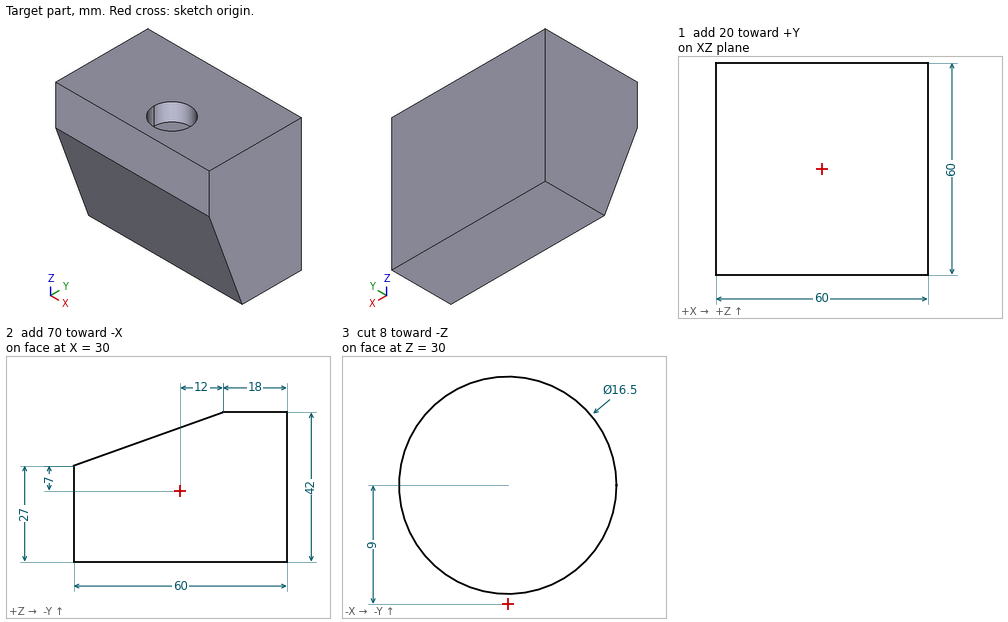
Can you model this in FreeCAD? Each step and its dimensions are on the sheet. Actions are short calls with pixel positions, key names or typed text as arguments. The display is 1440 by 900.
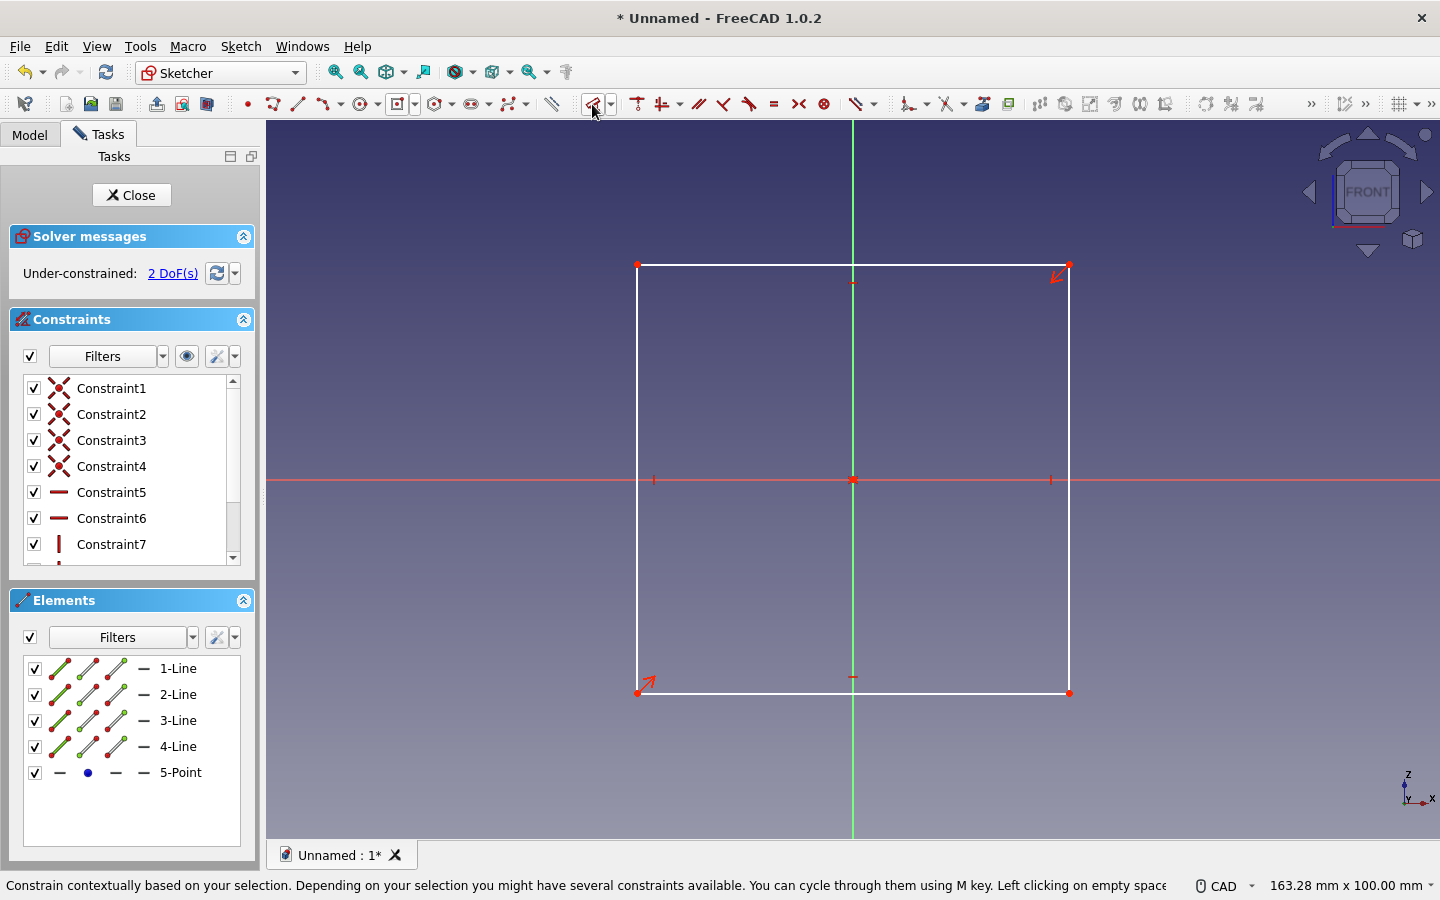
click(767, 694)
click(754, 728)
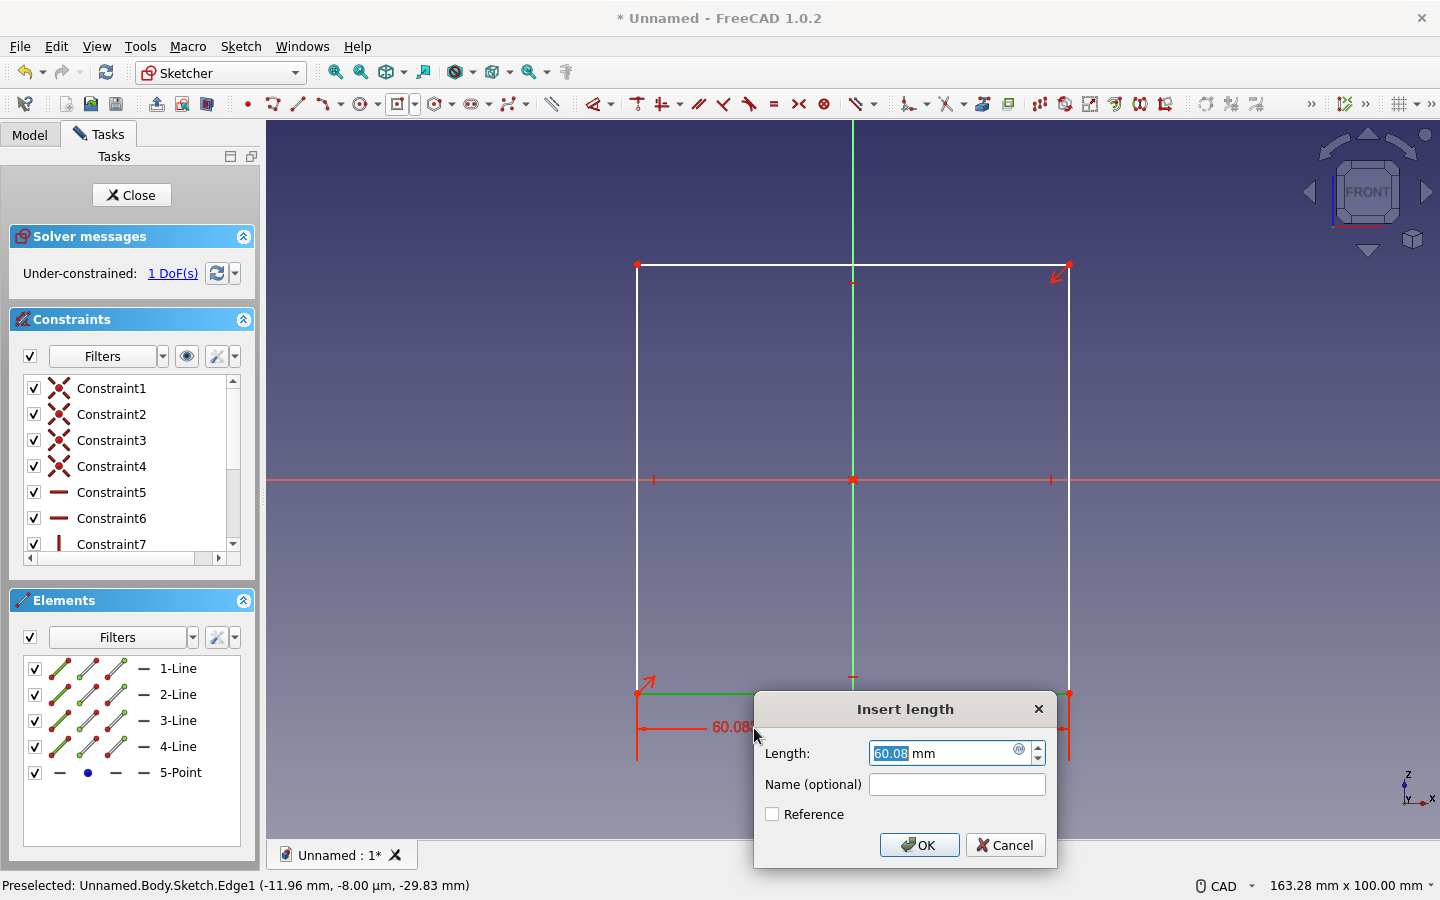
text(60)
key(Return)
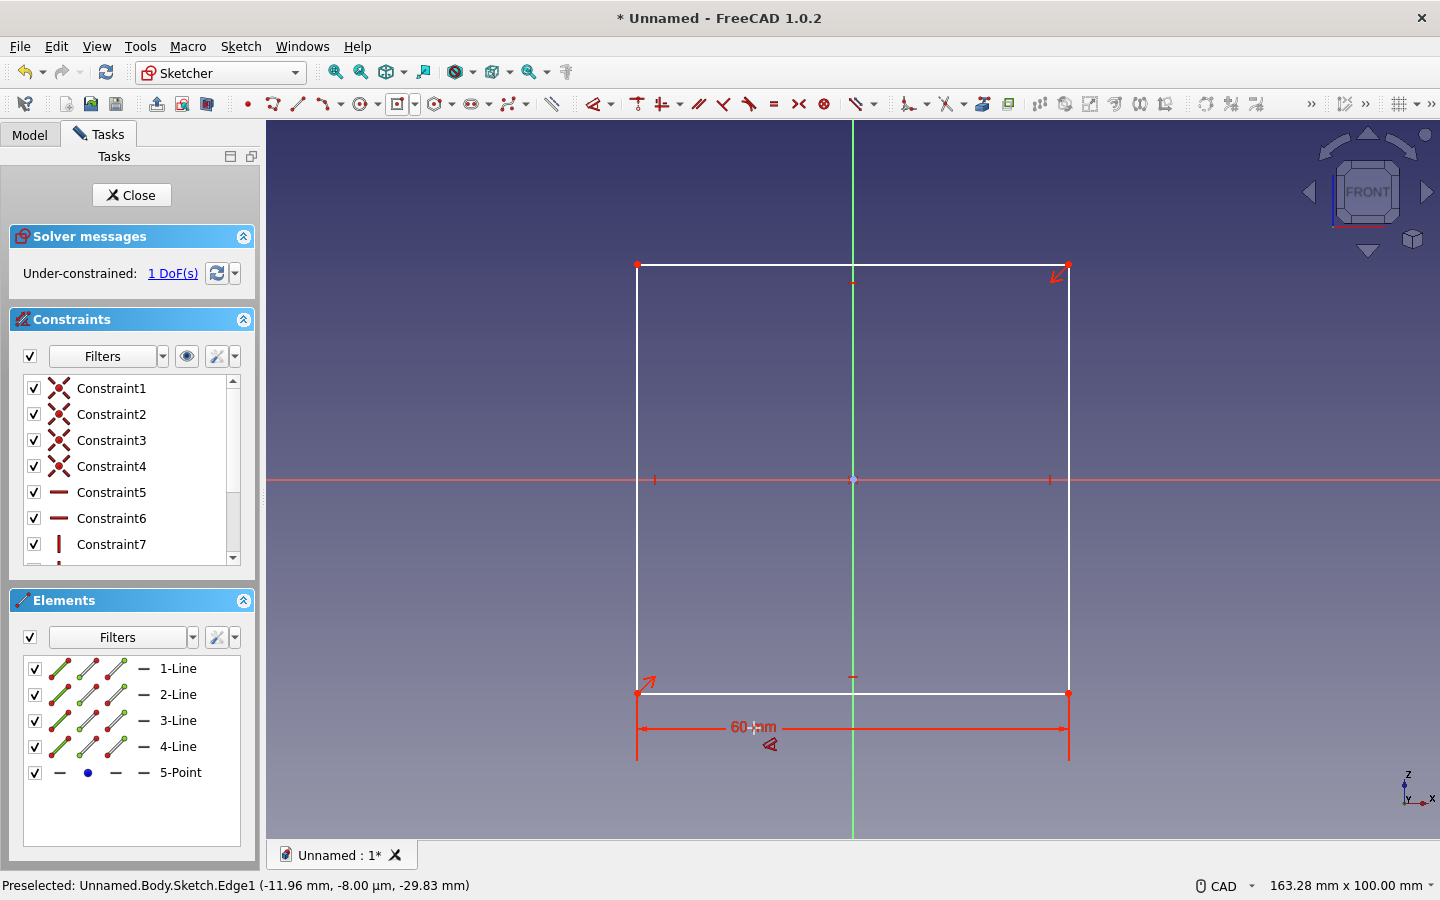
click(1069, 565)
click(1103, 381)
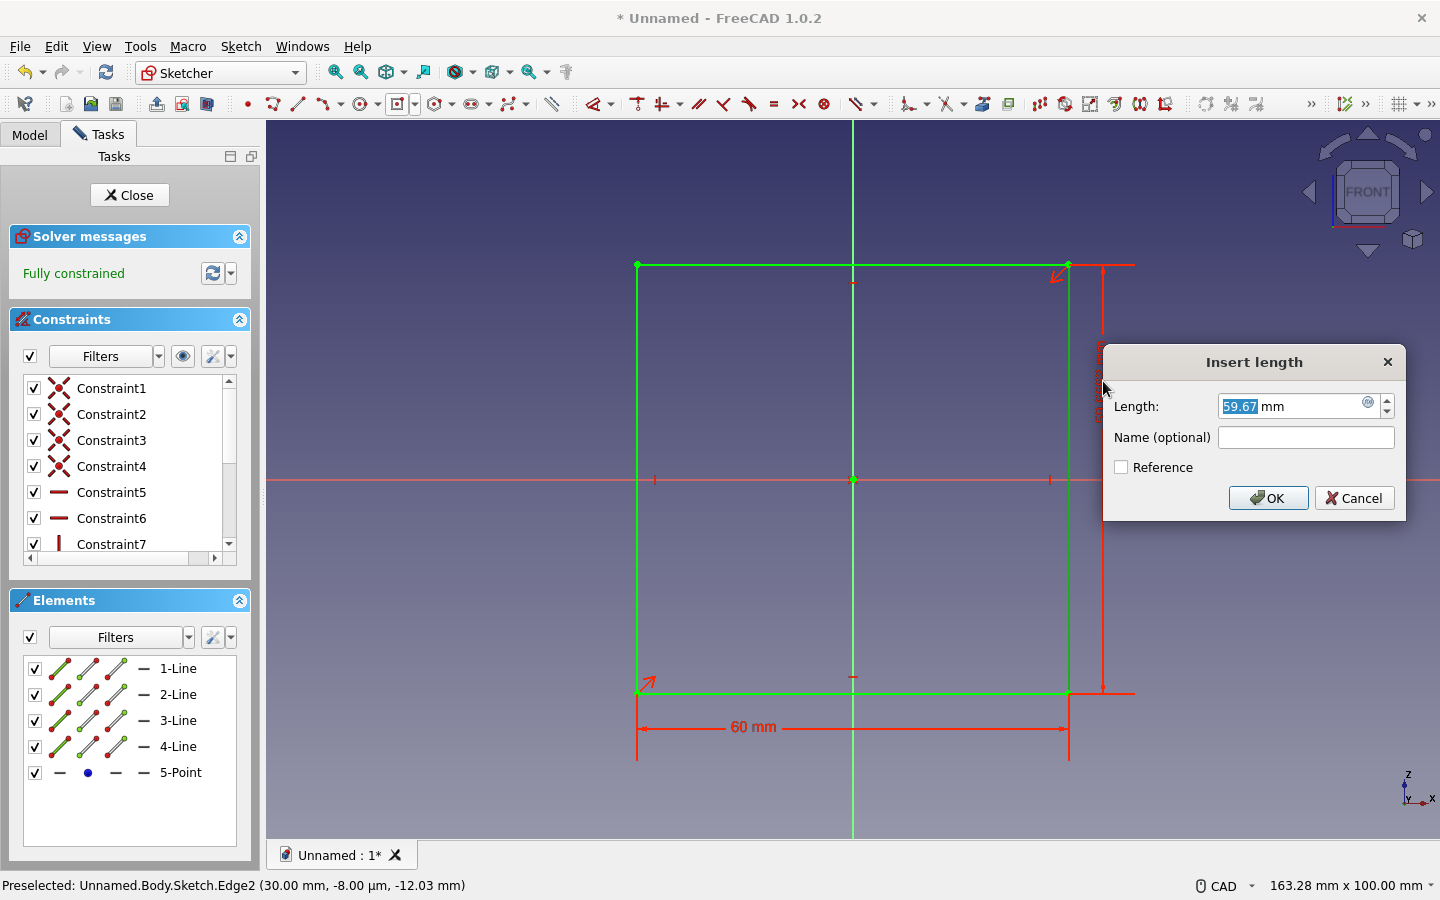
text(60)
key(Return)
key(Escape)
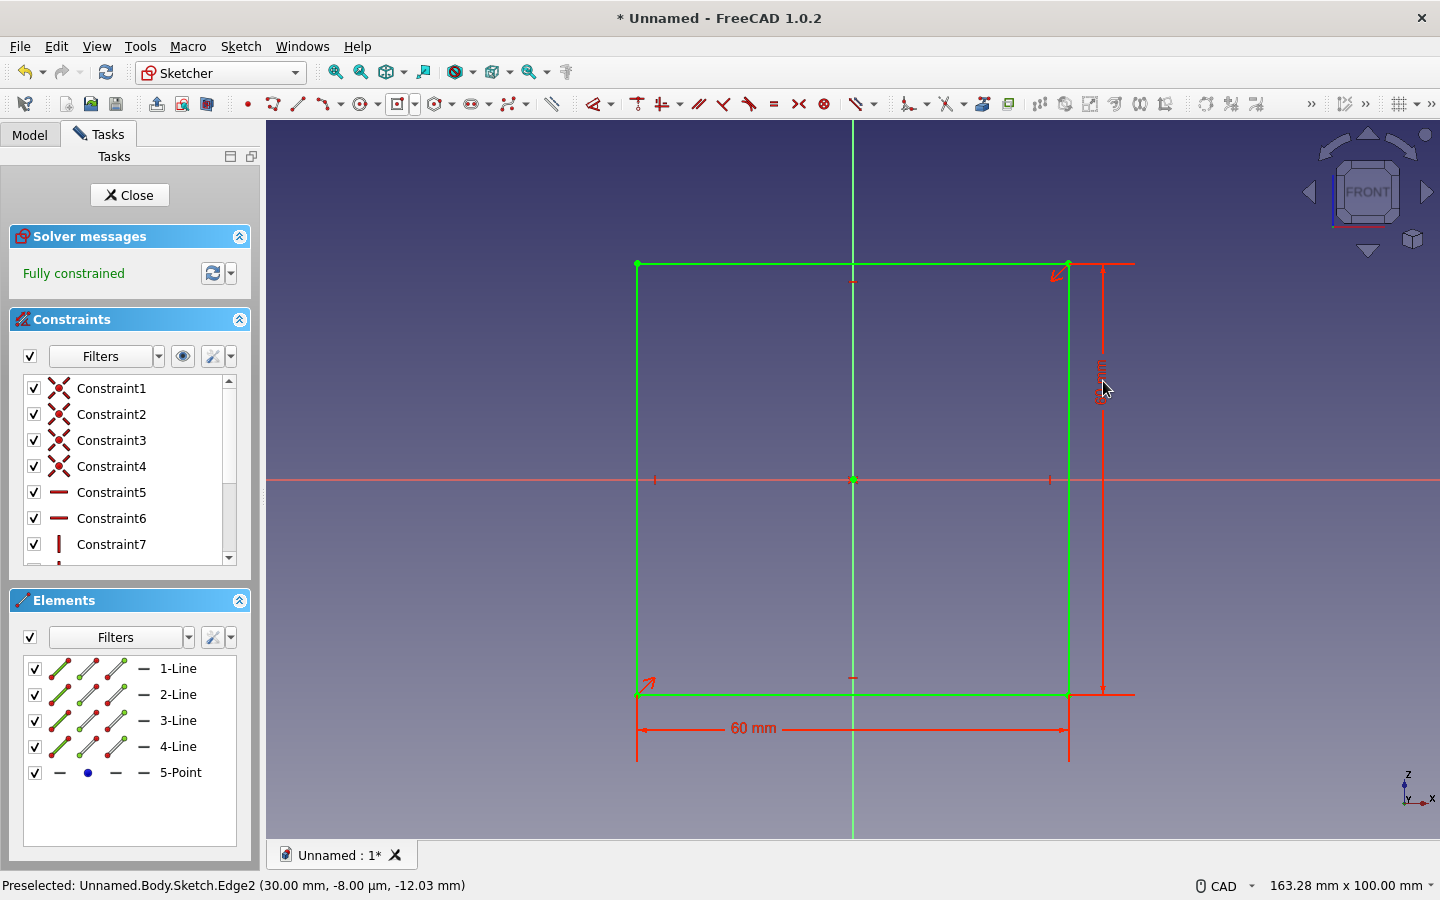
click(130, 195)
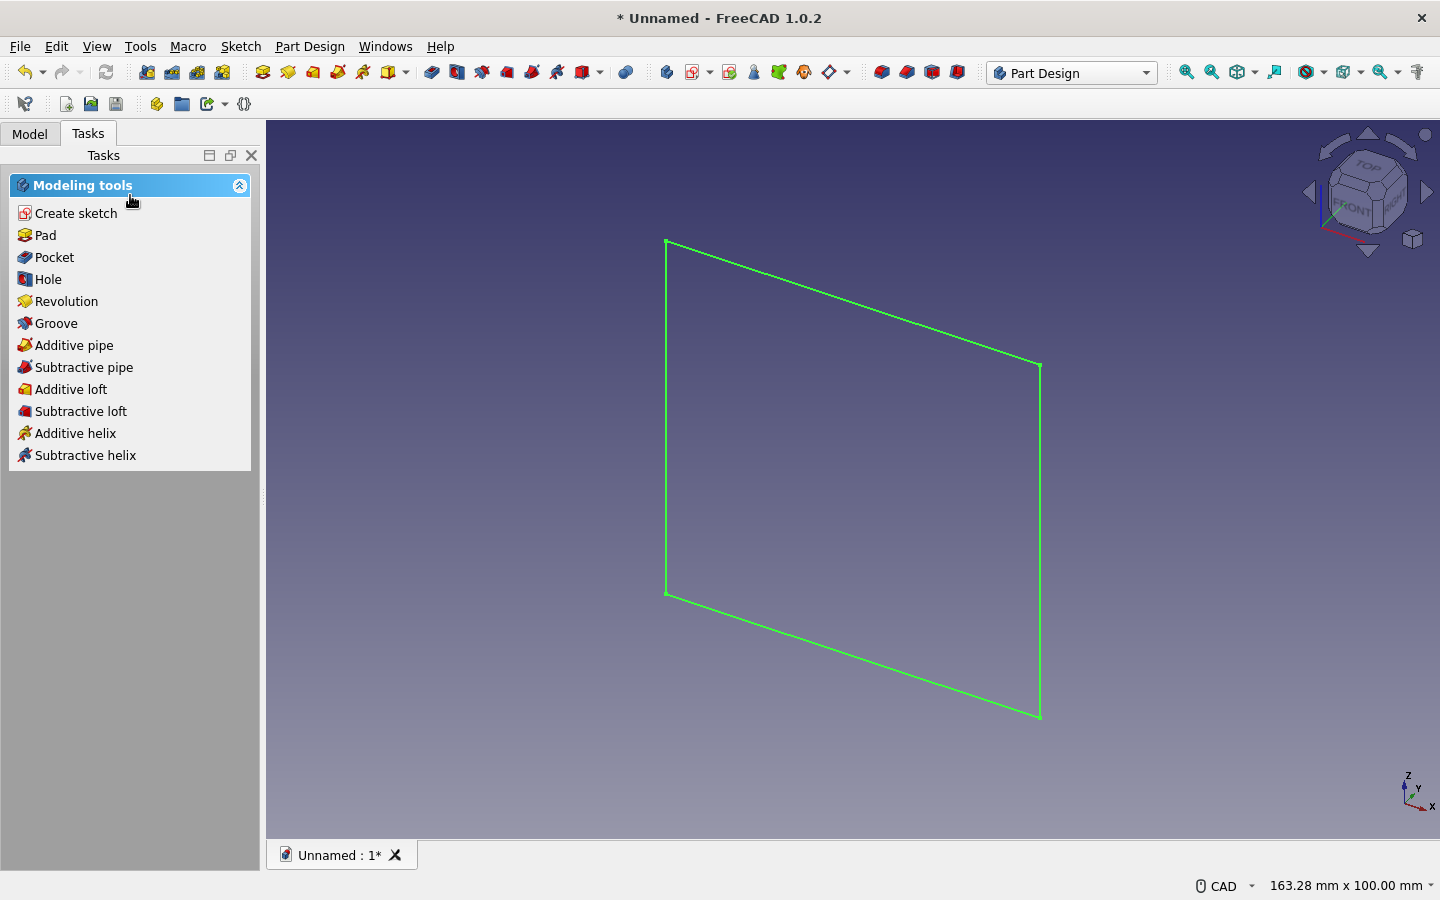
click(263, 72)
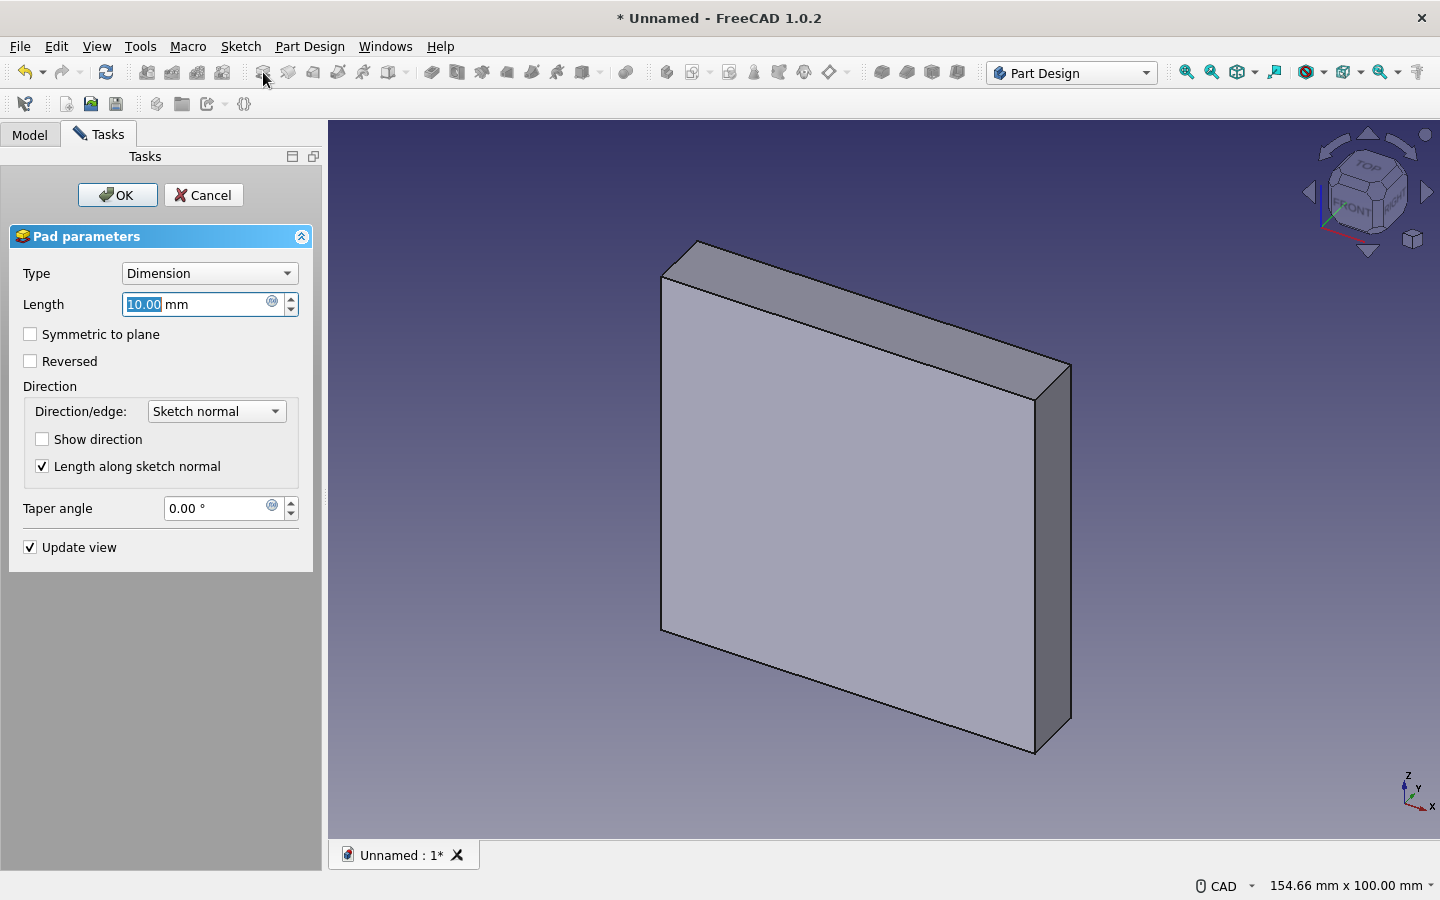
text(20)
key(Tab)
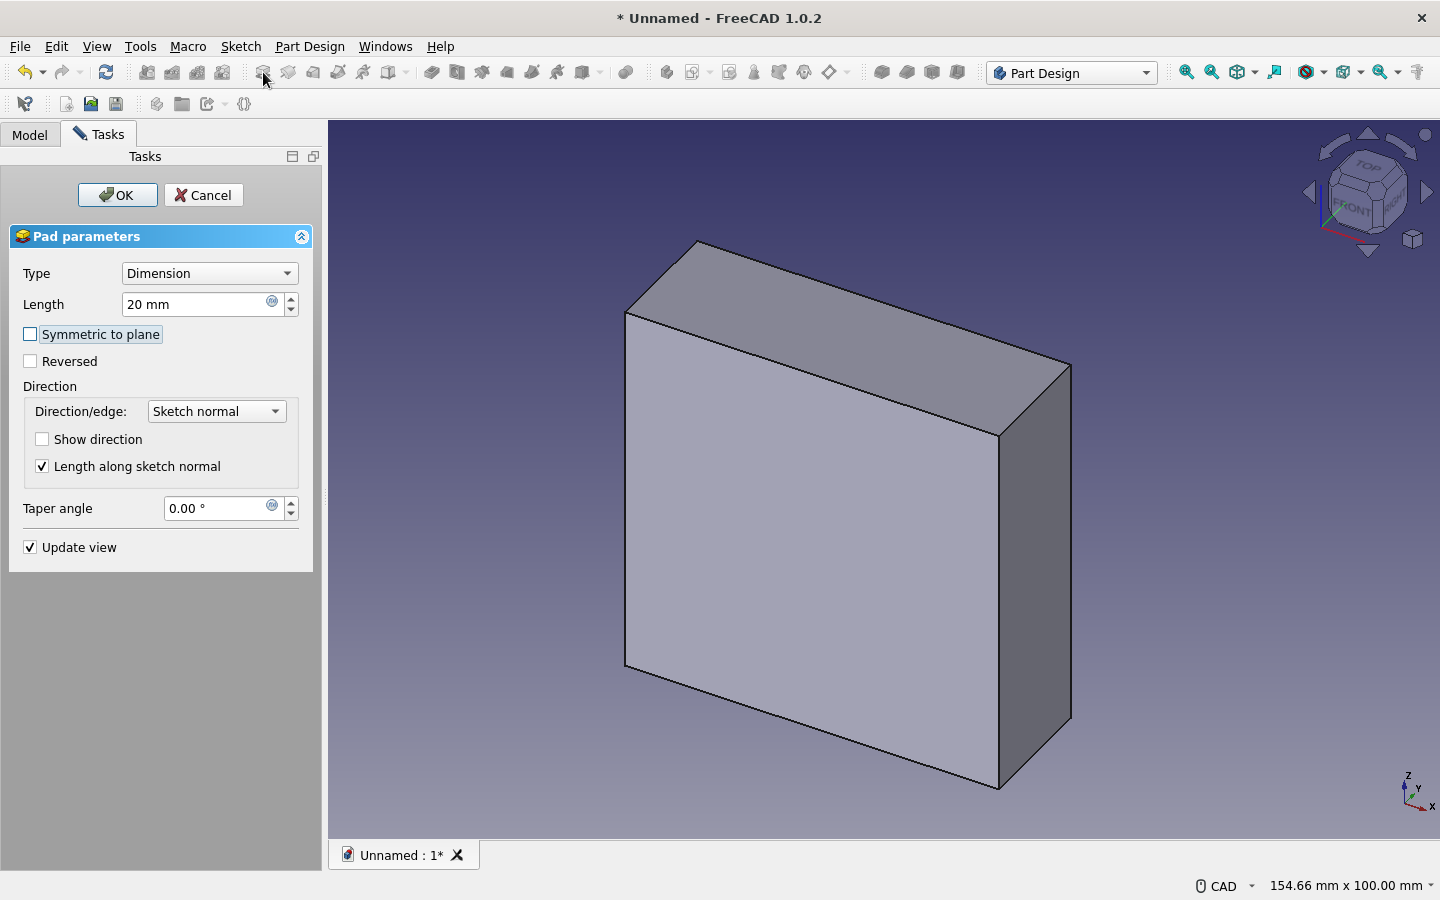
click(31, 361)